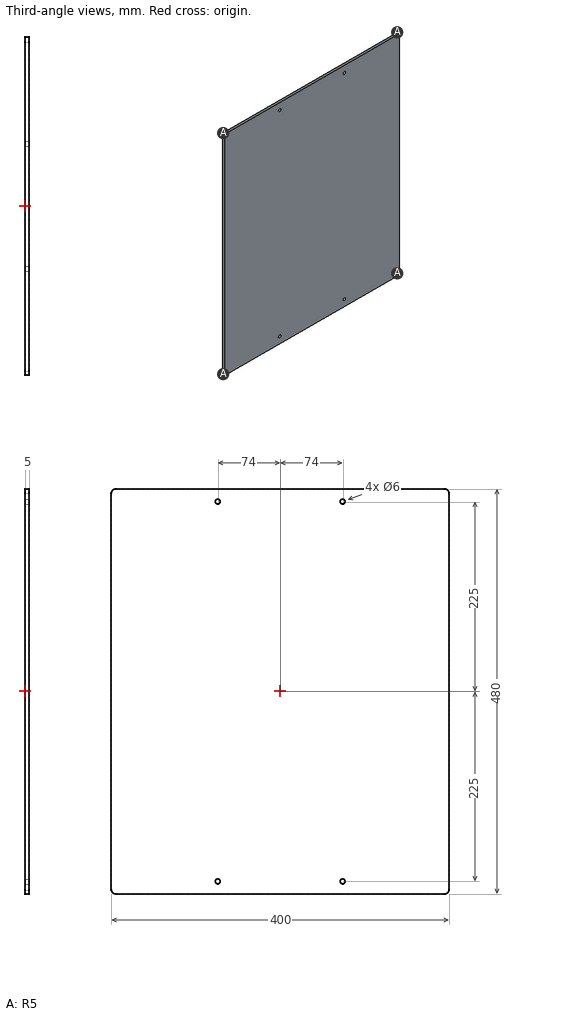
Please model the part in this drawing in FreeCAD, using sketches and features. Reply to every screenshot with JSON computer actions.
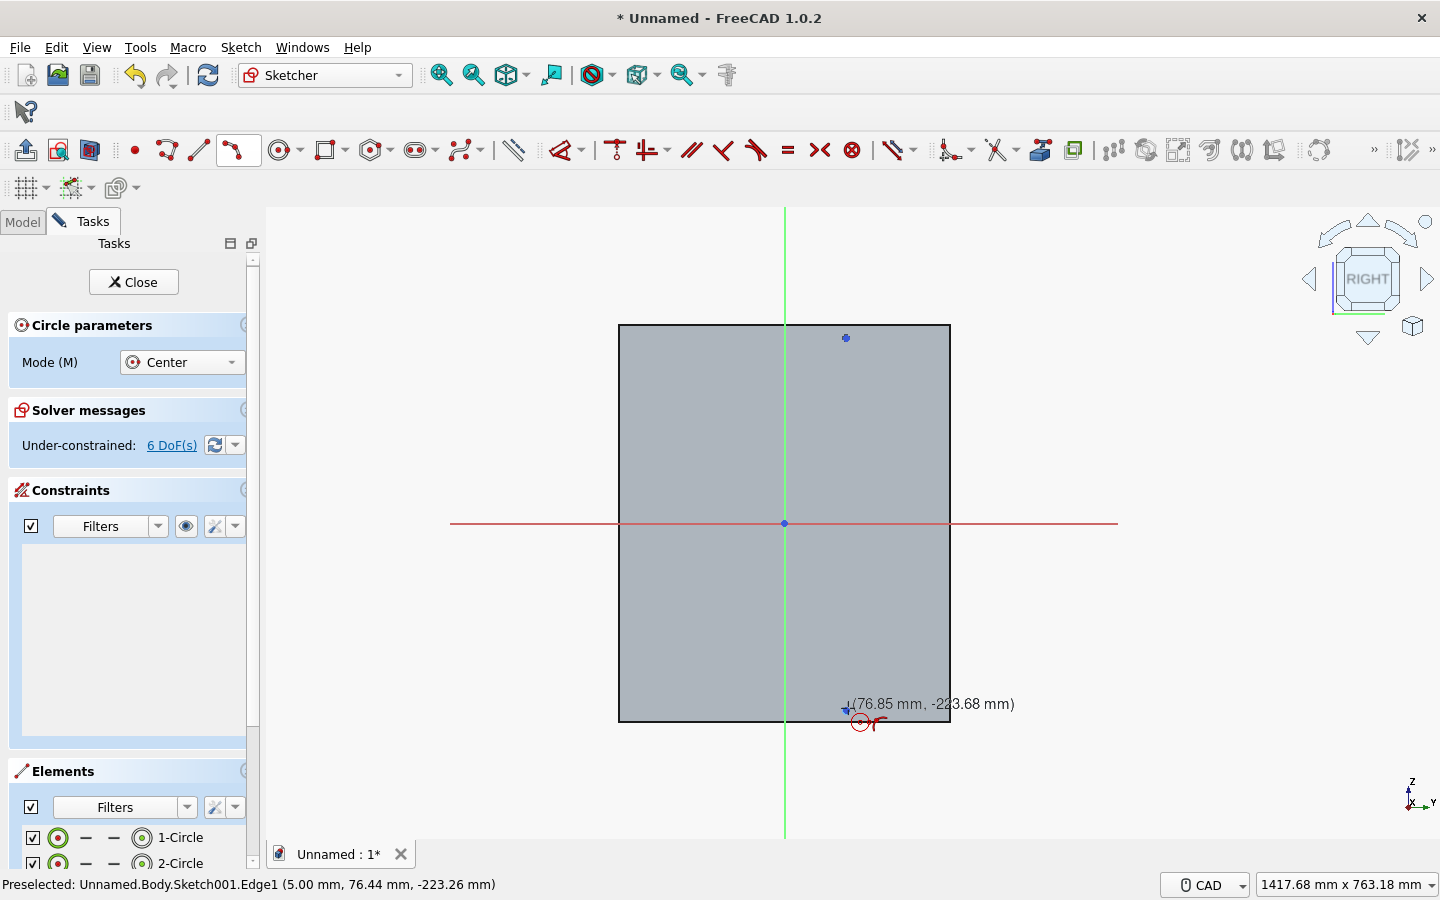
{"action": "scroll", "coordinate": [724, 337], "scroll_direction": "up", "scroll_amount": 12}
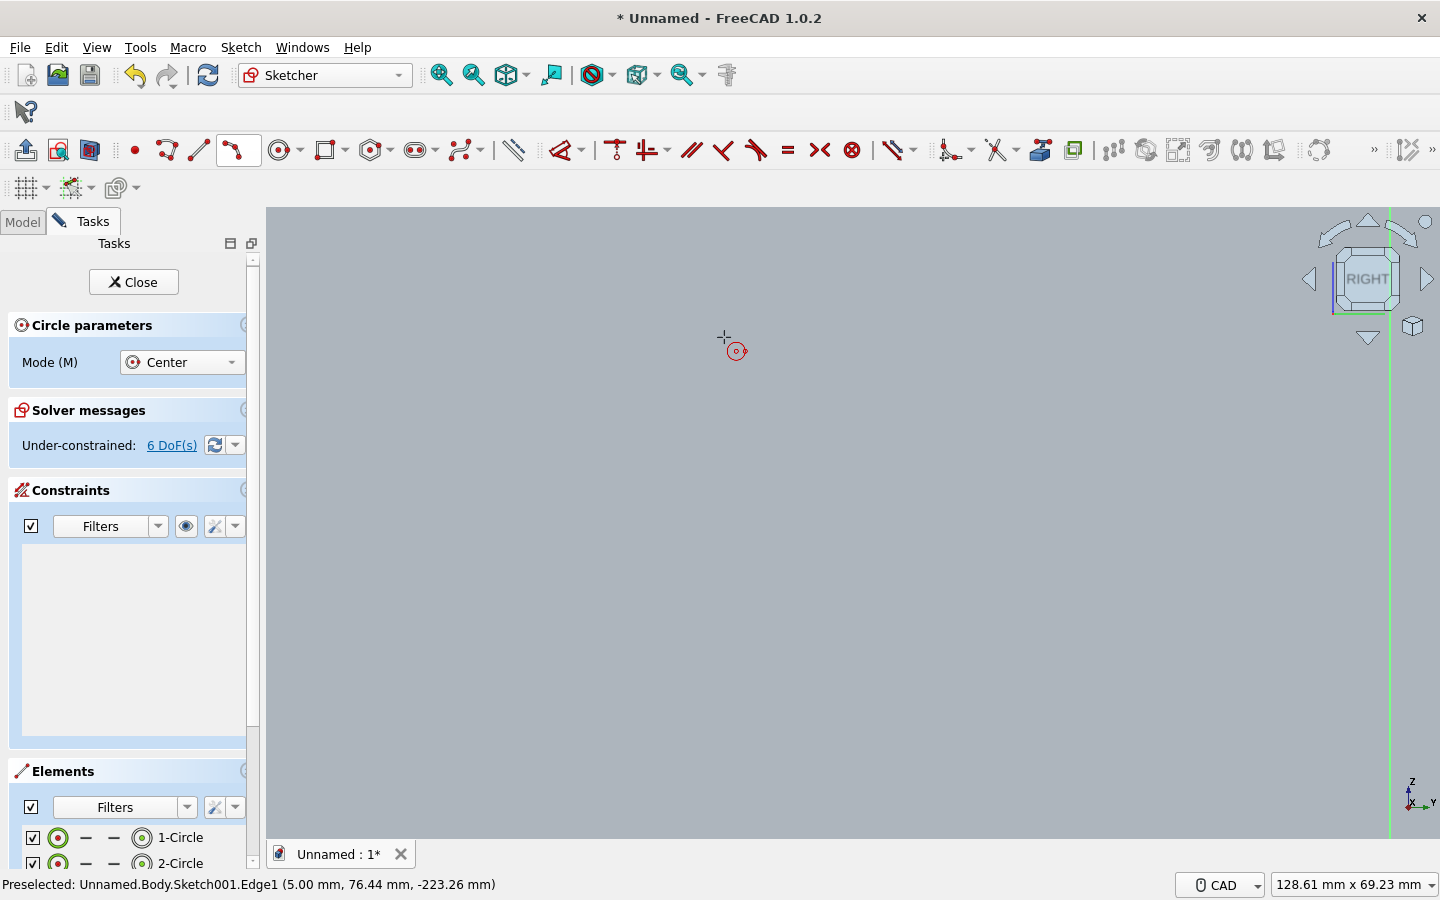
{"action": "scroll", "coordinate": [724, 337], "scroll_direction": "down", "scroll_amount": 12}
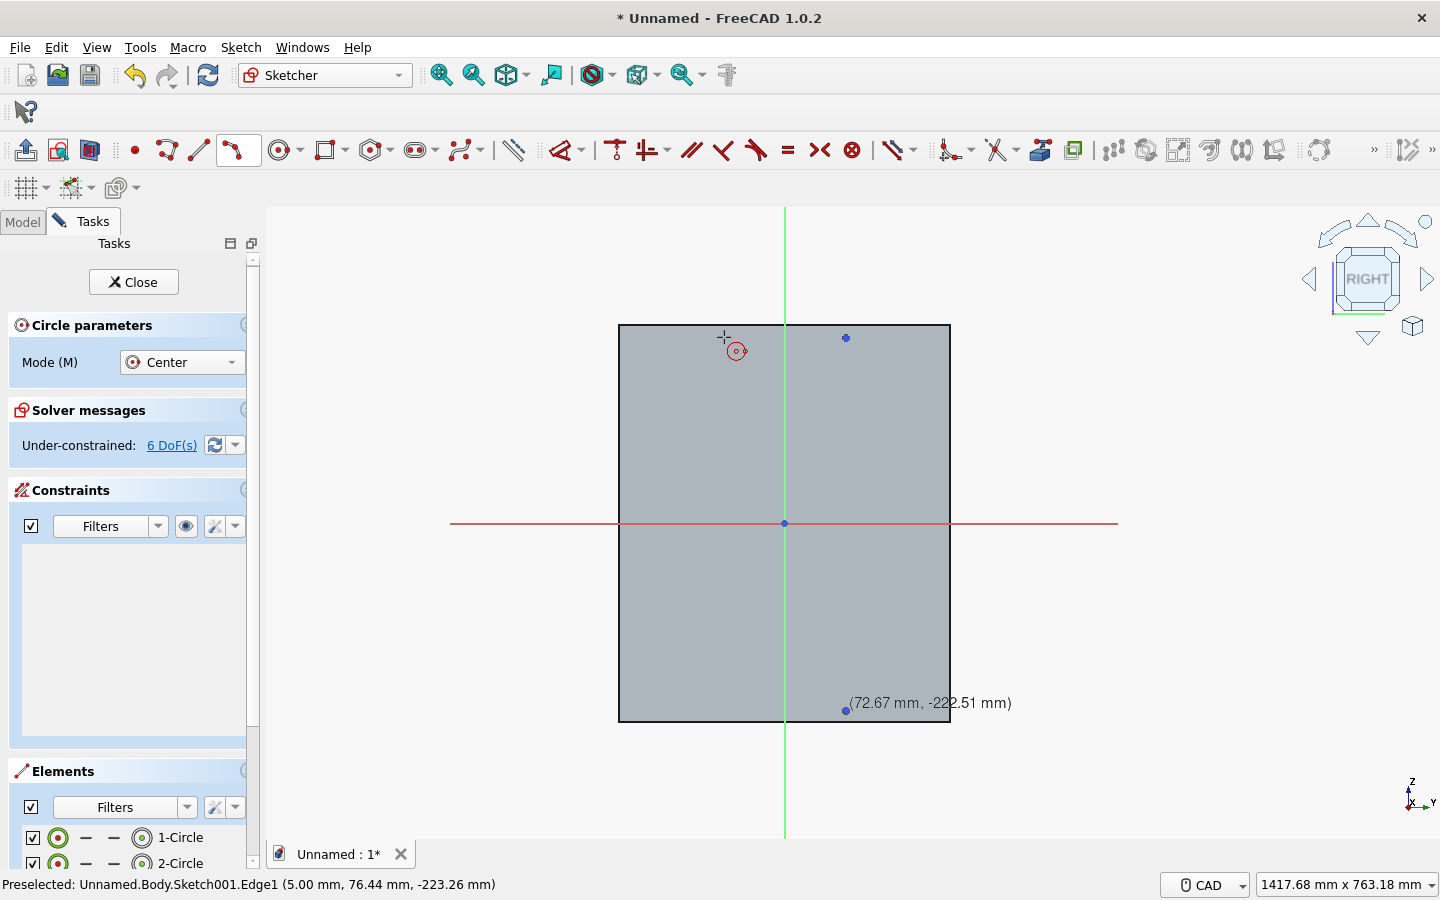
{"action": "left_click", "coordinate": [724, 337]}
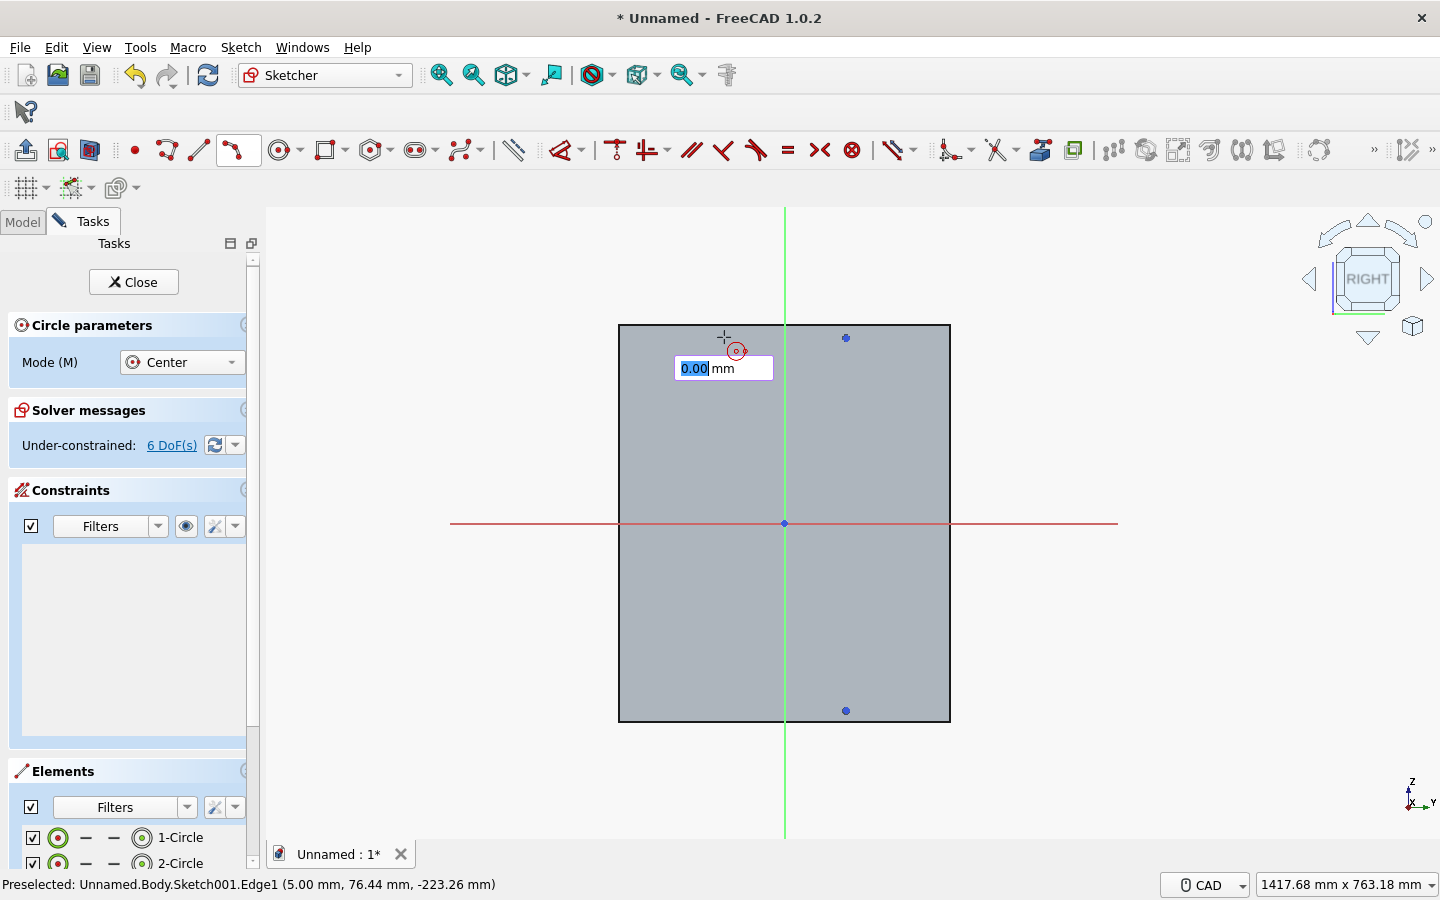
{"action": "scroll", "coordinate": [725, 336], "scroll_direction": "up", "scroll_amount": 10}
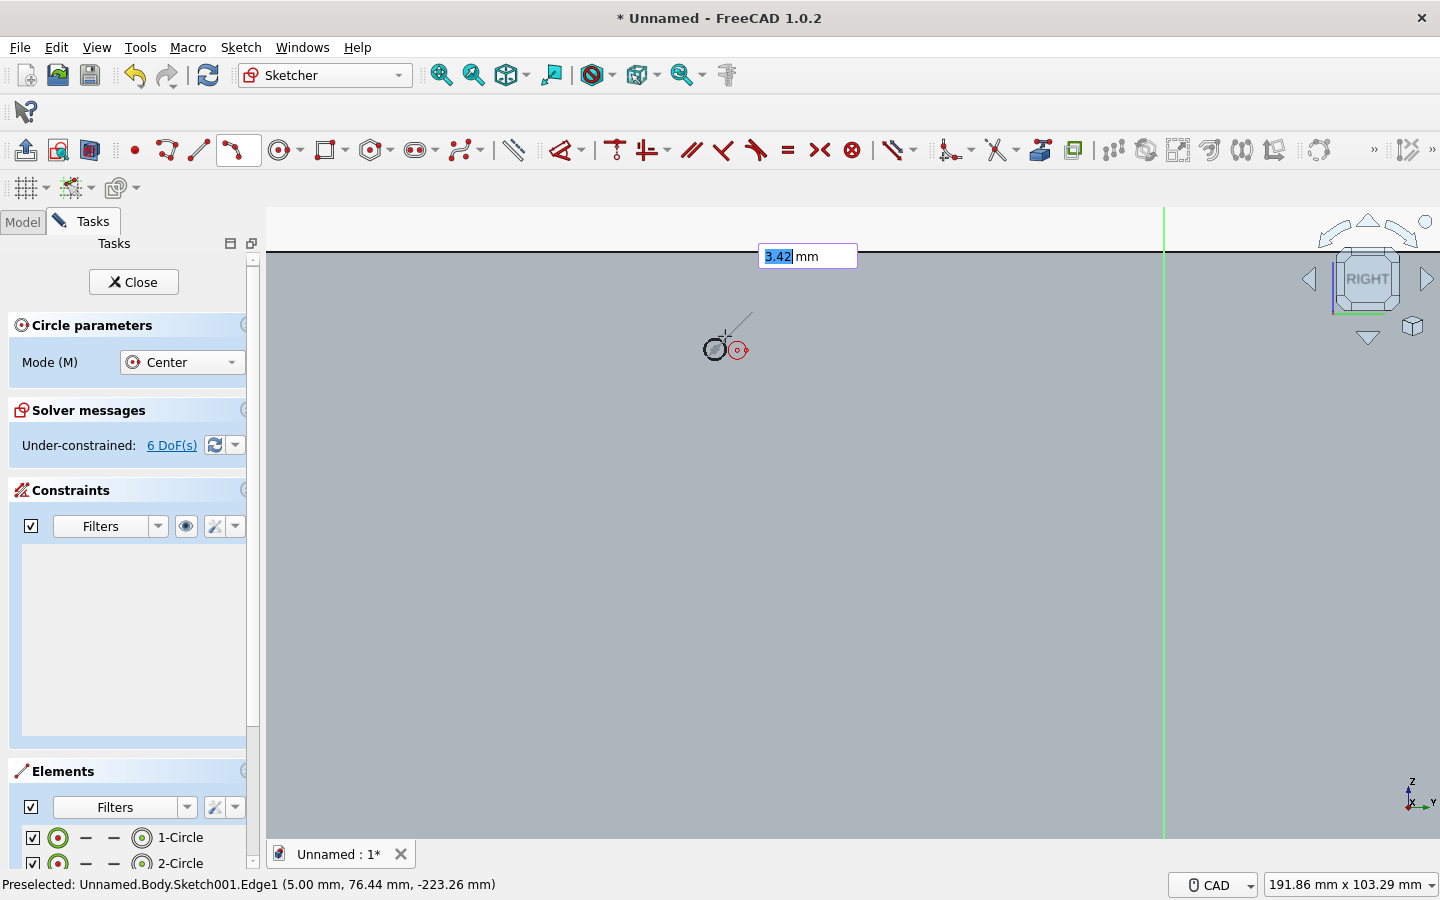
{"action": "left_click", "coordinate": [724, 331]}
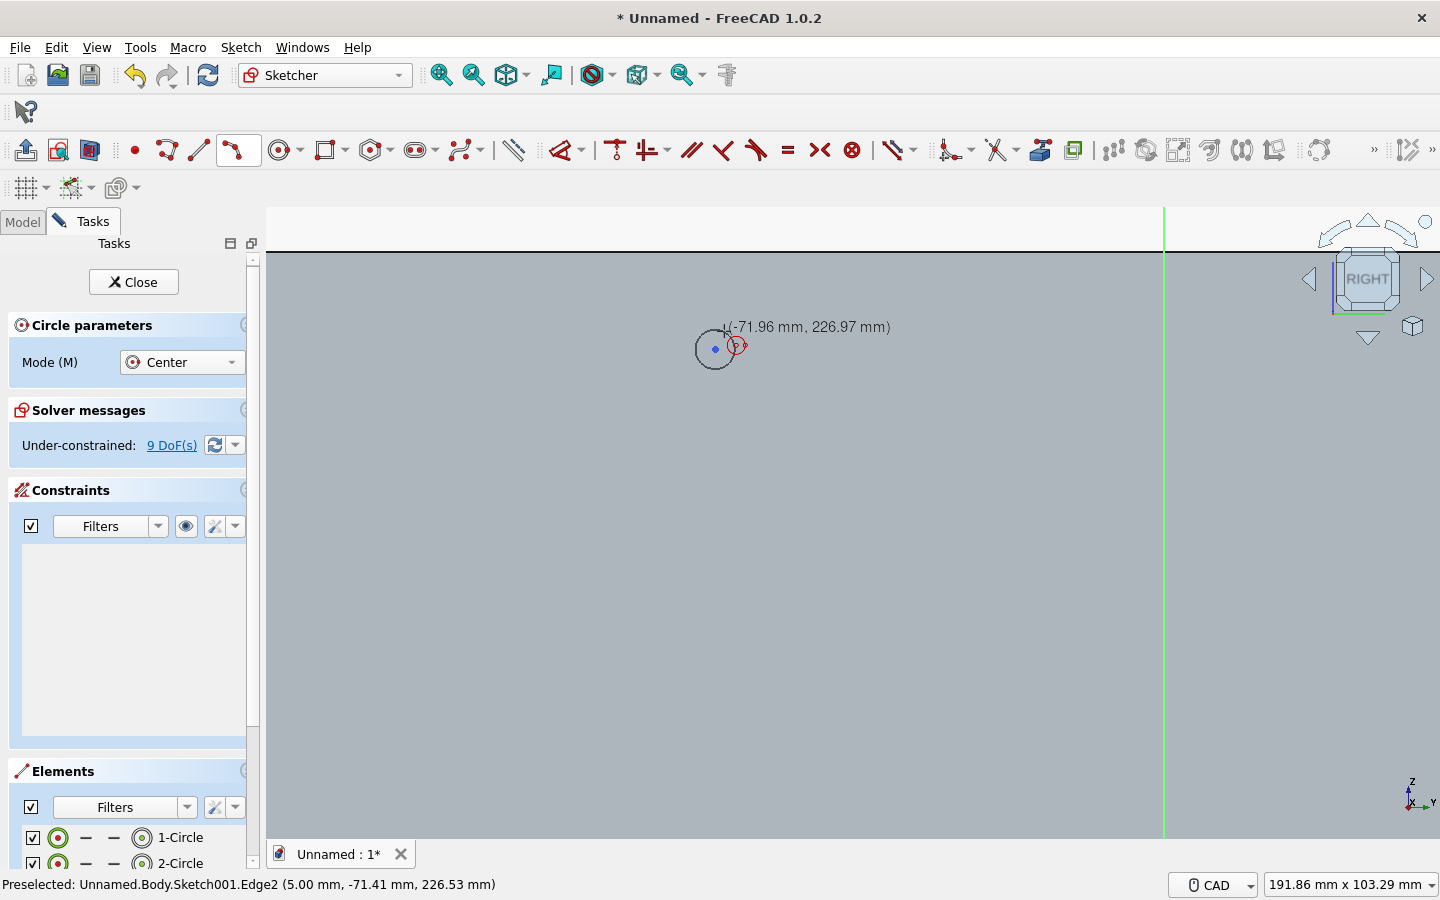
{"action": "scroll", "coordinate": [725, 336], "scroll_direction": "down", "scroll_amount": 10}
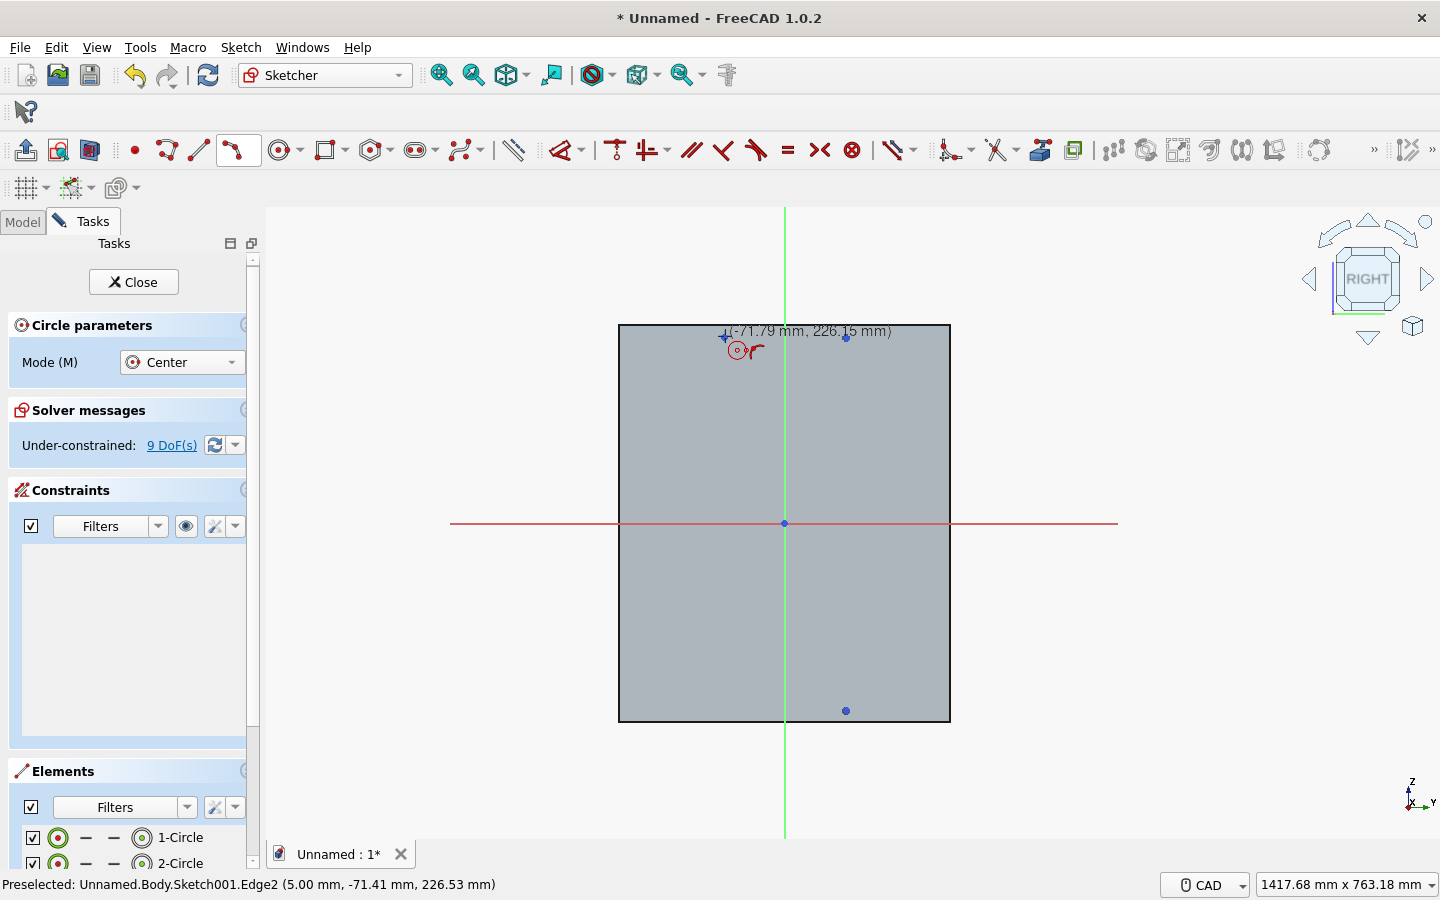
{"action": "scroll", "coordinate": [724, 710], "scroll_direction": "up", "scroll_amount": 12}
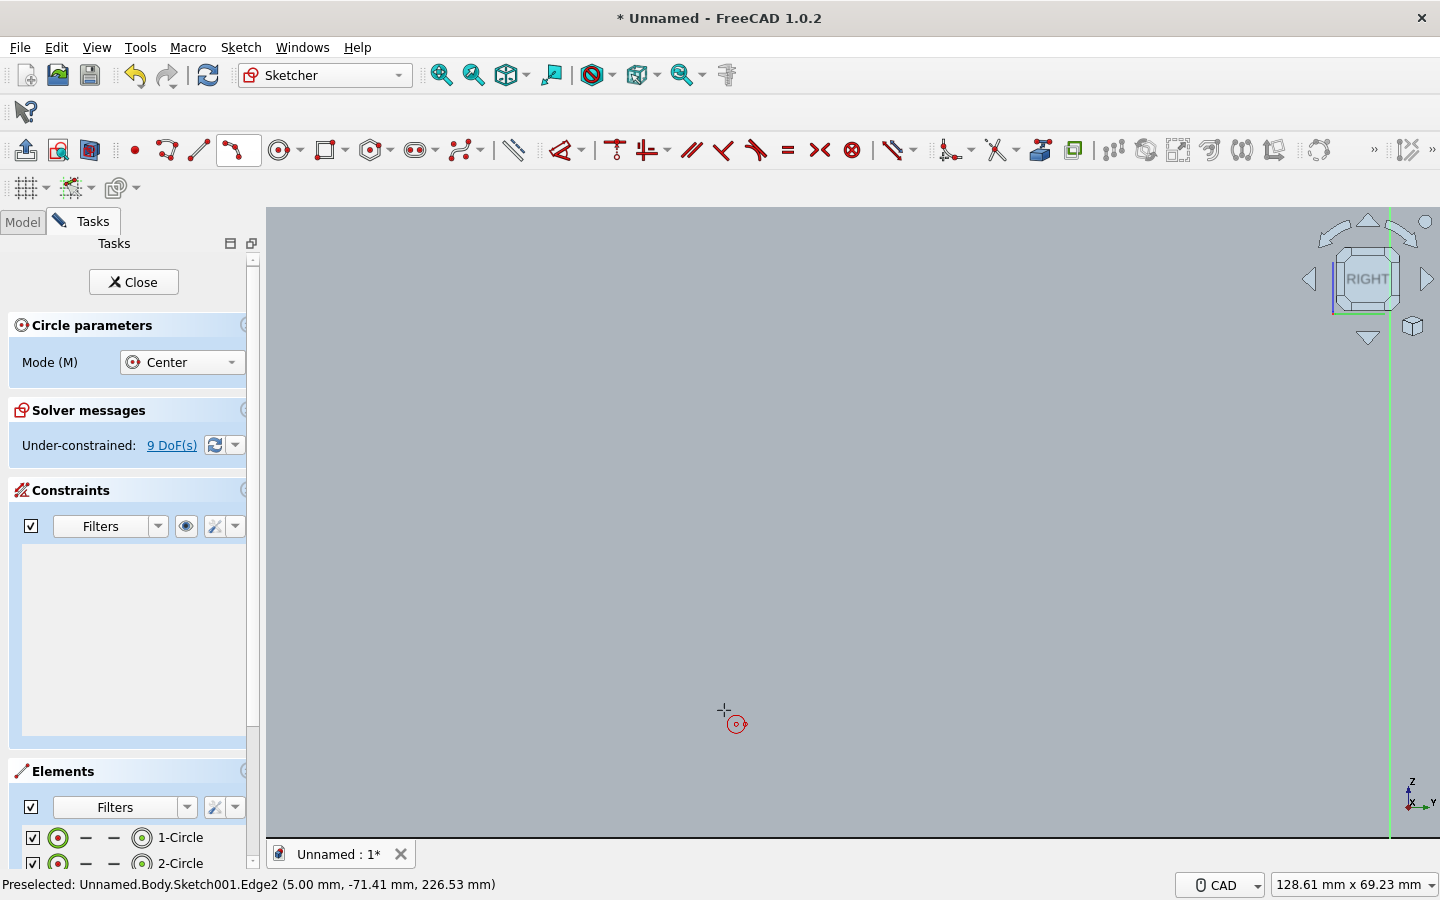
{"action": "scroll", "coordinate": [724, 710], "scroll_direction": "down", "scroll_amount": 12}